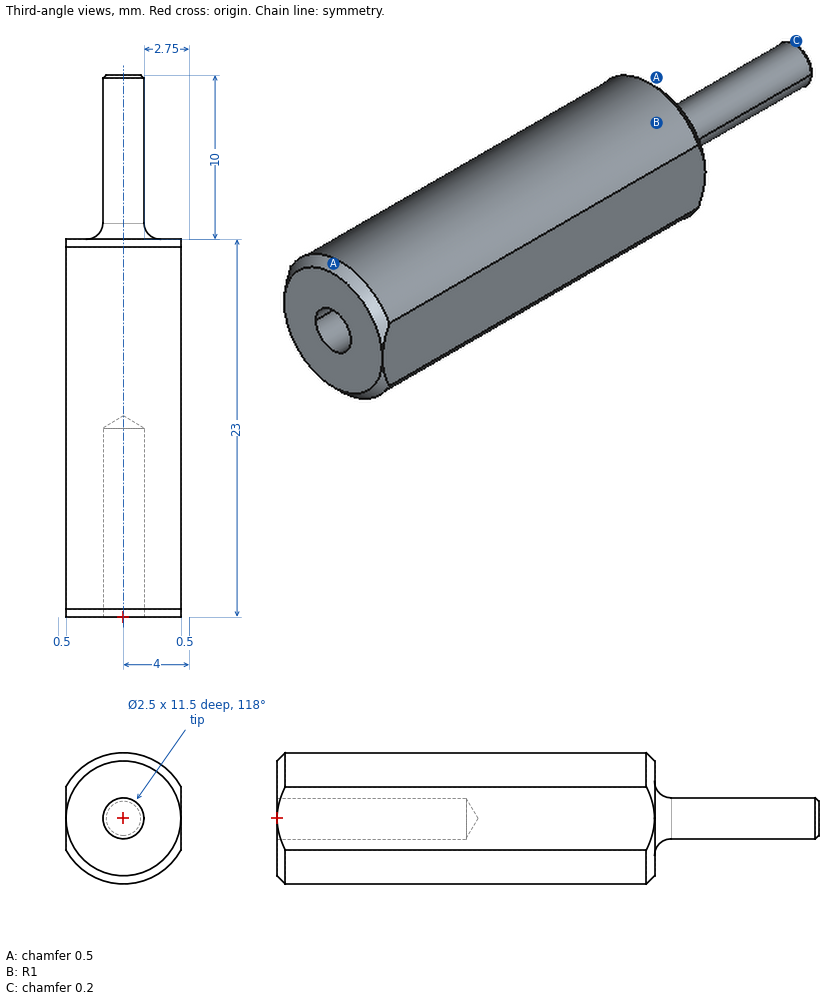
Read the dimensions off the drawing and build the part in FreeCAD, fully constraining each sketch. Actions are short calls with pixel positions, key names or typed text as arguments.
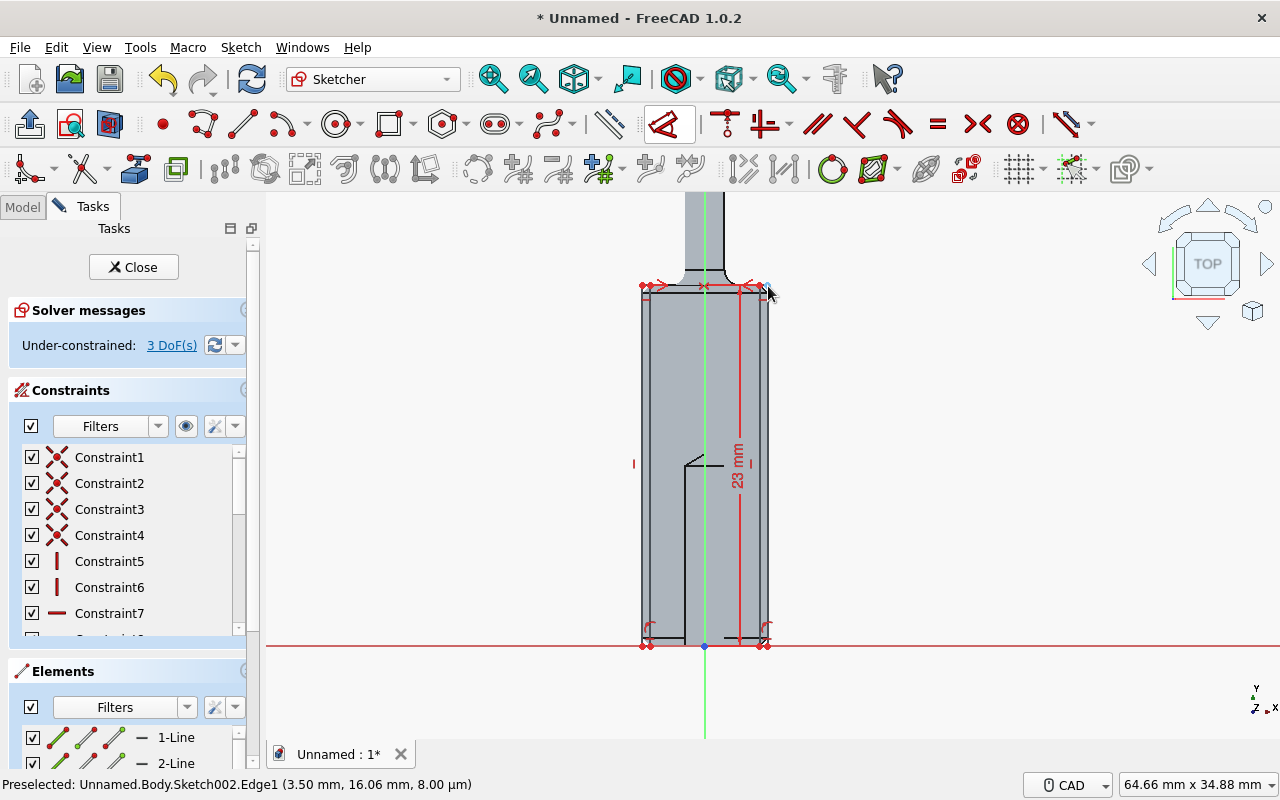
scroll(768, 646, up, 3)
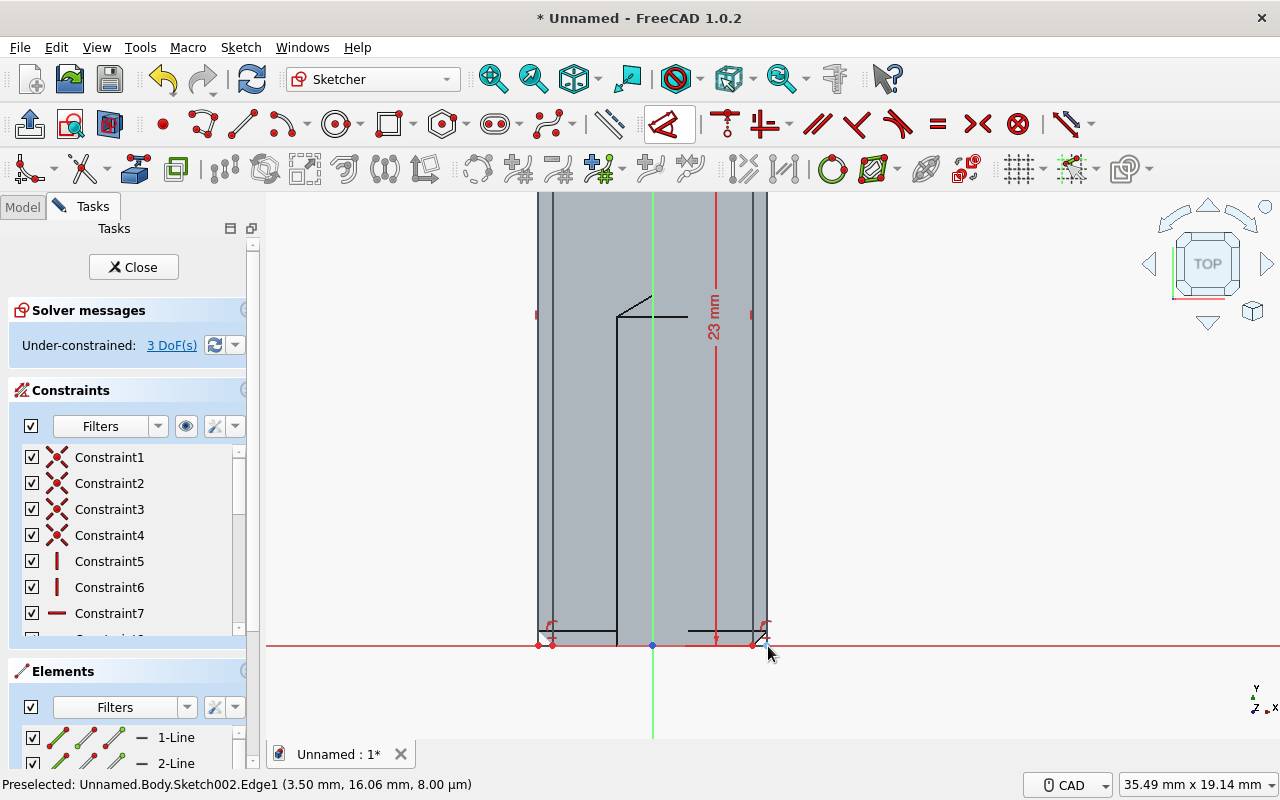
click(767, 646)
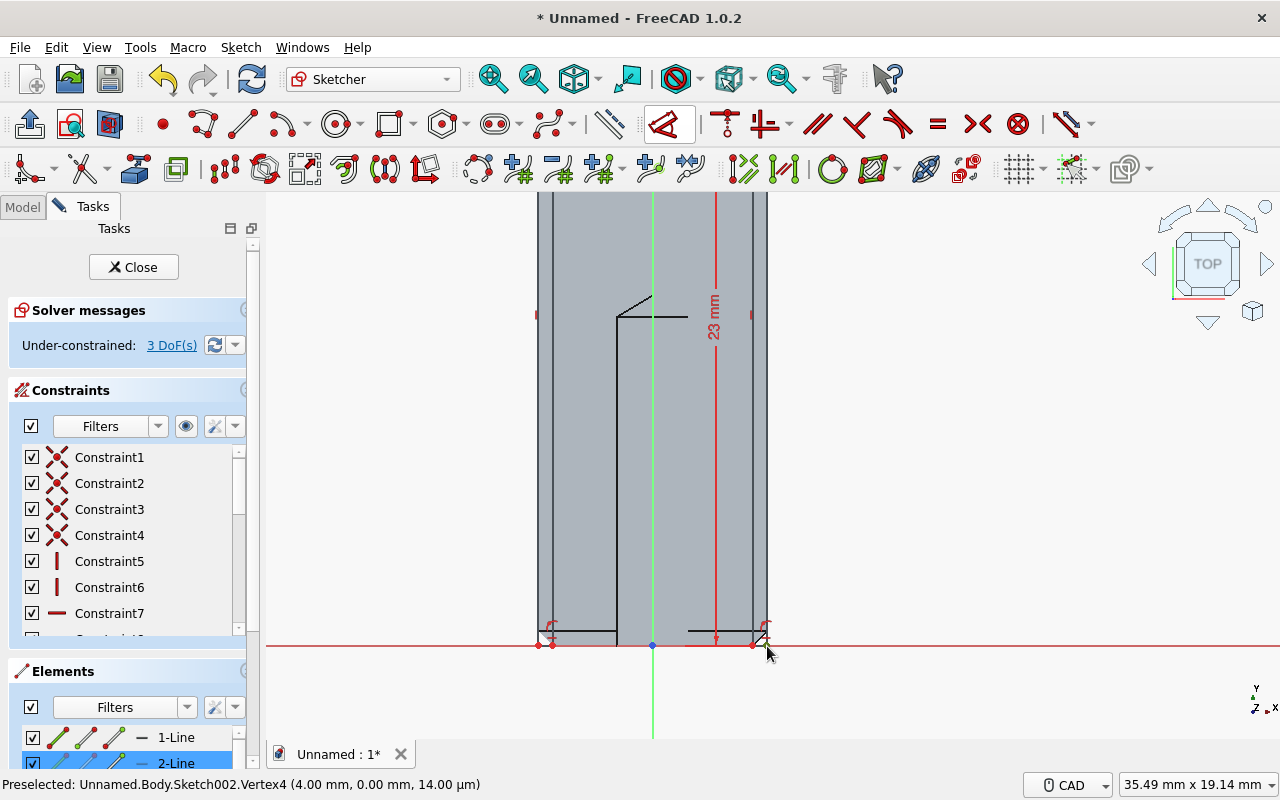
key(l)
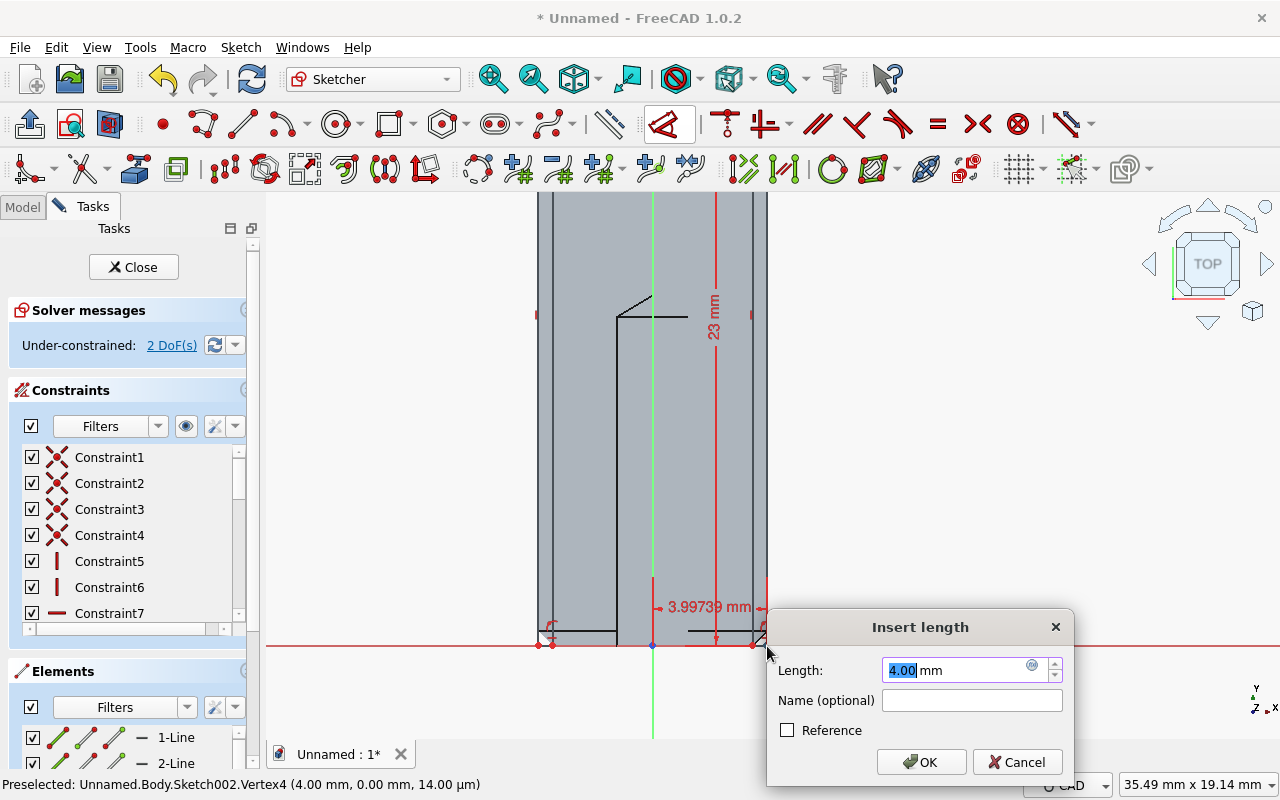
text(4)
key(Return)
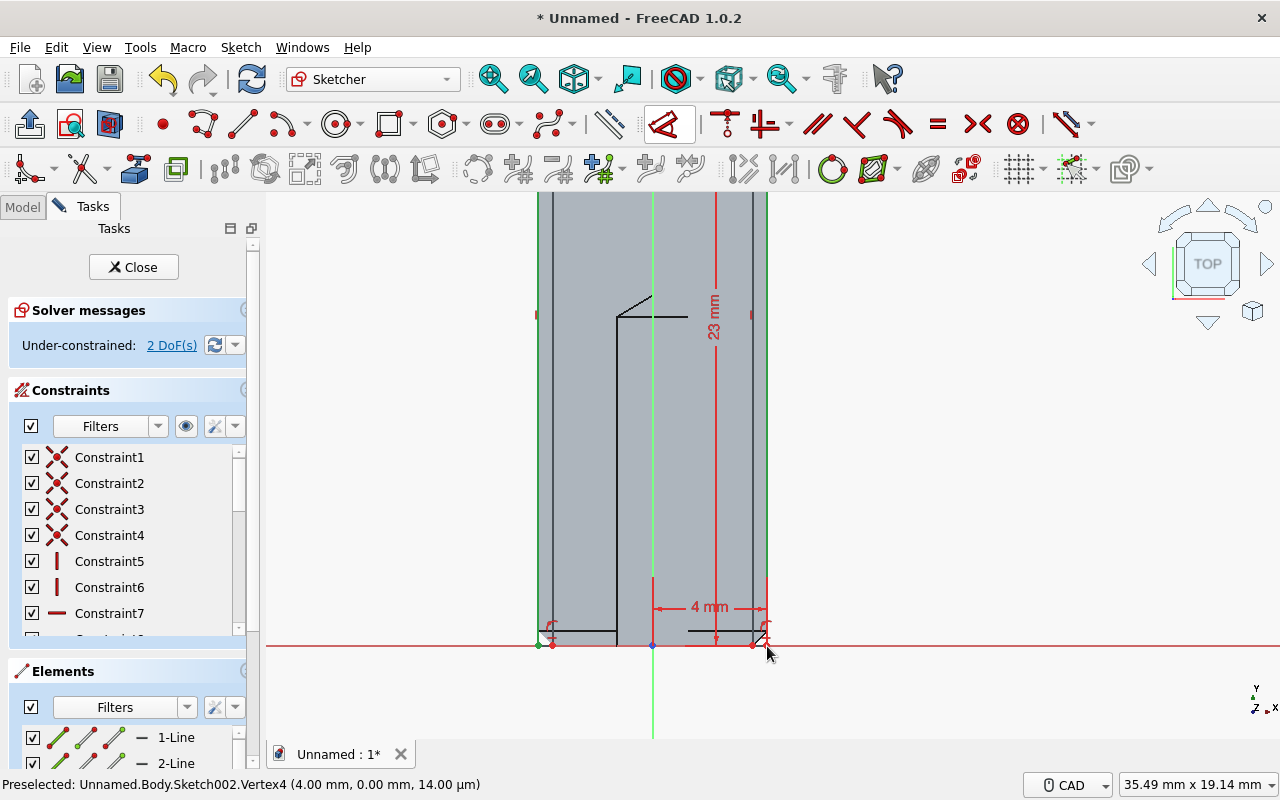
scroll(760, 646, up, 6)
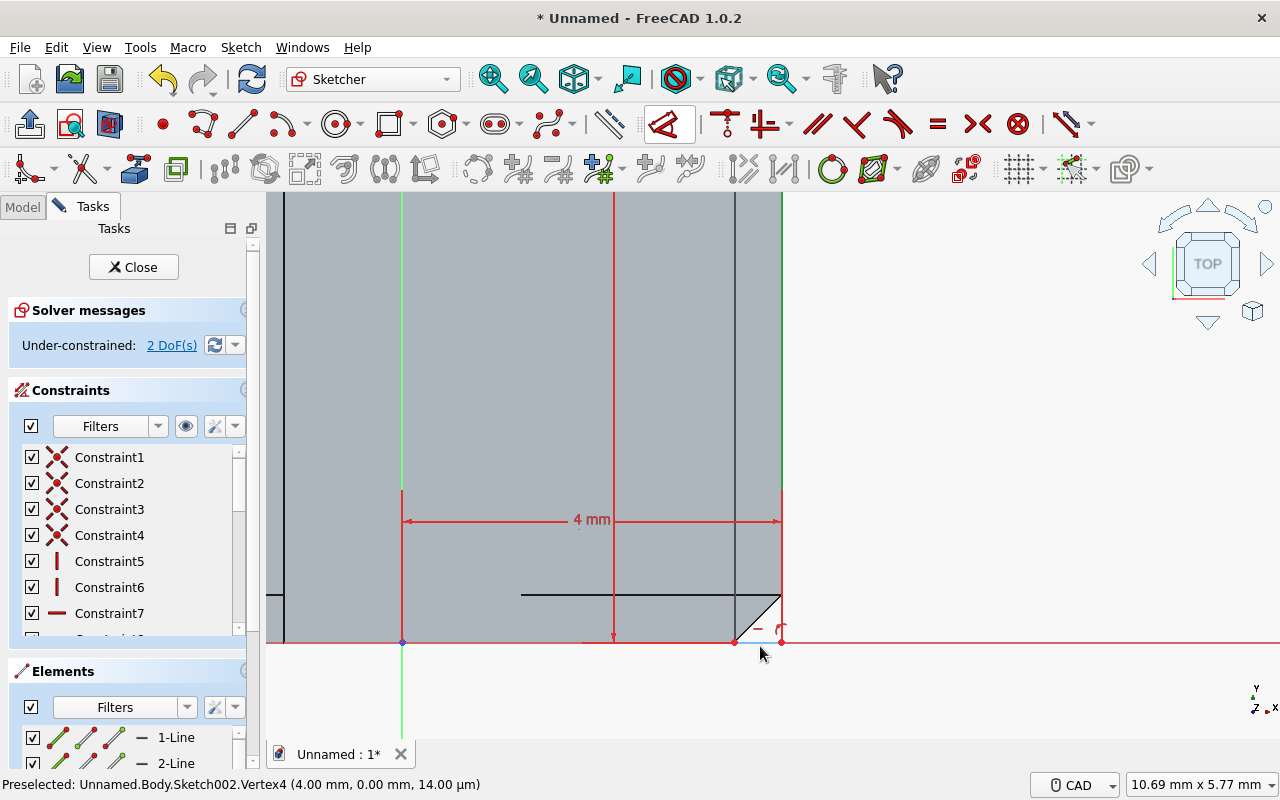
click(758, 643)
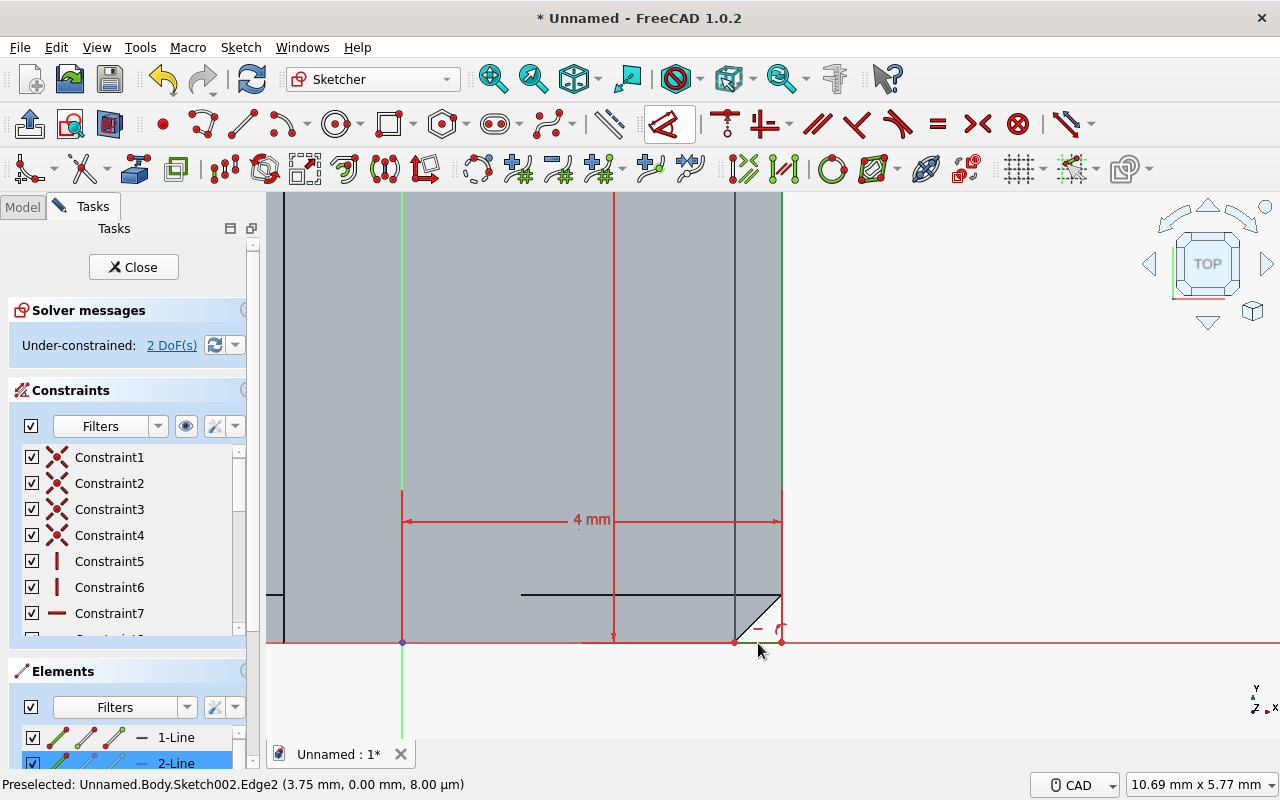
key(l)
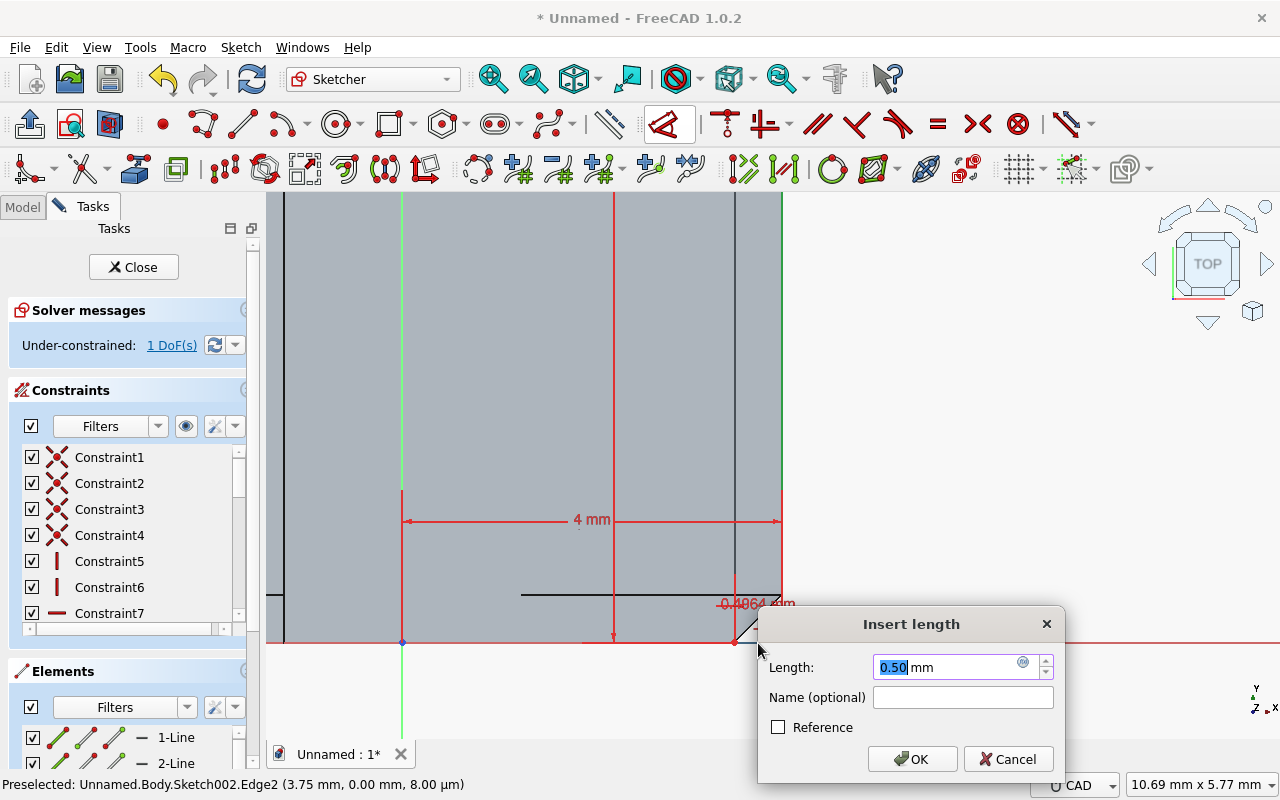
text(0.5)
key(Return)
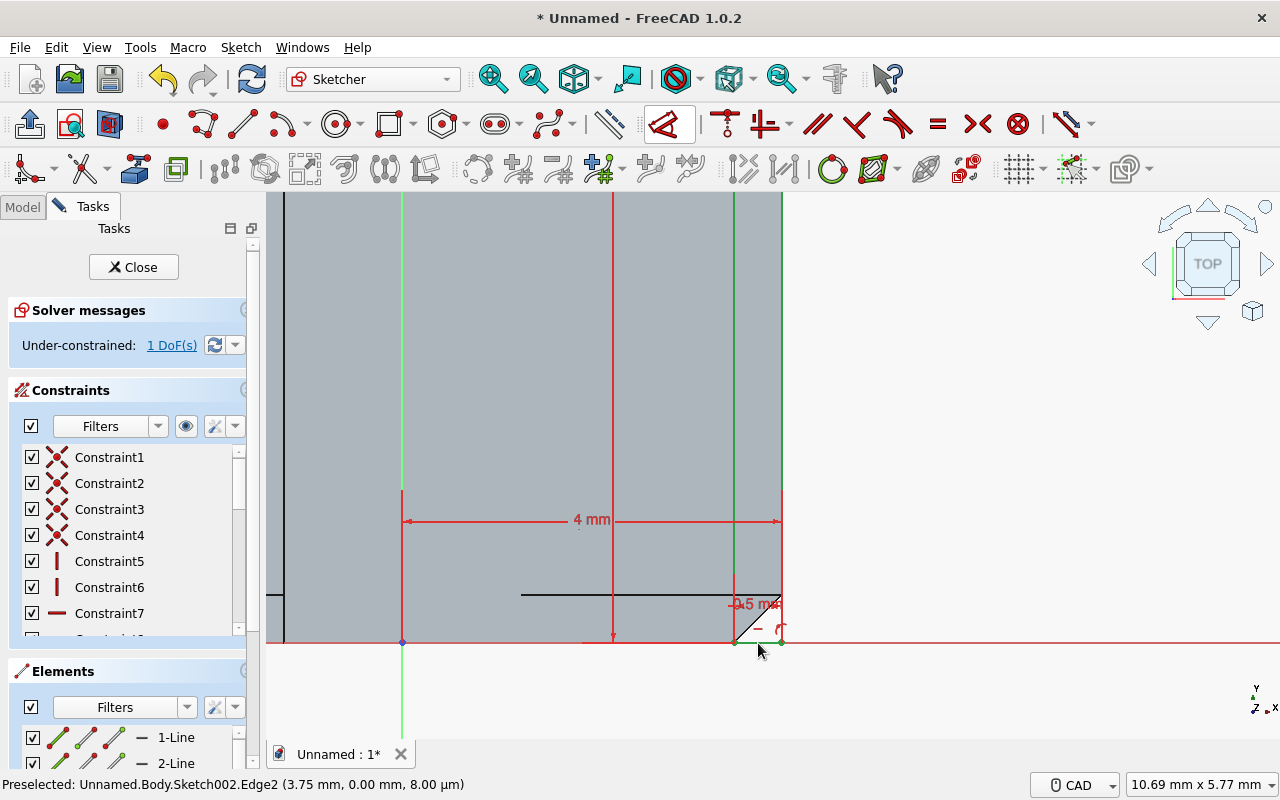
scroll(764, 646, down, 9)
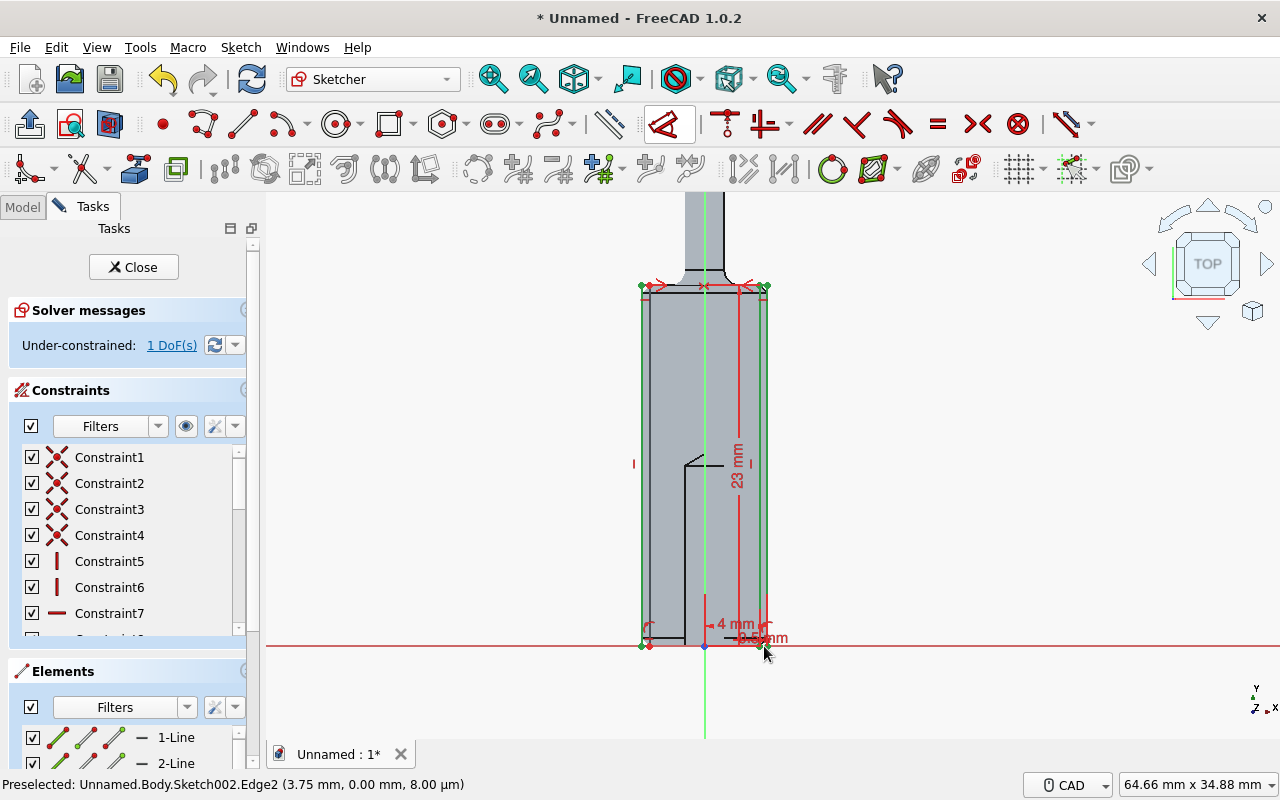
scroll(644, 646, up, 9)